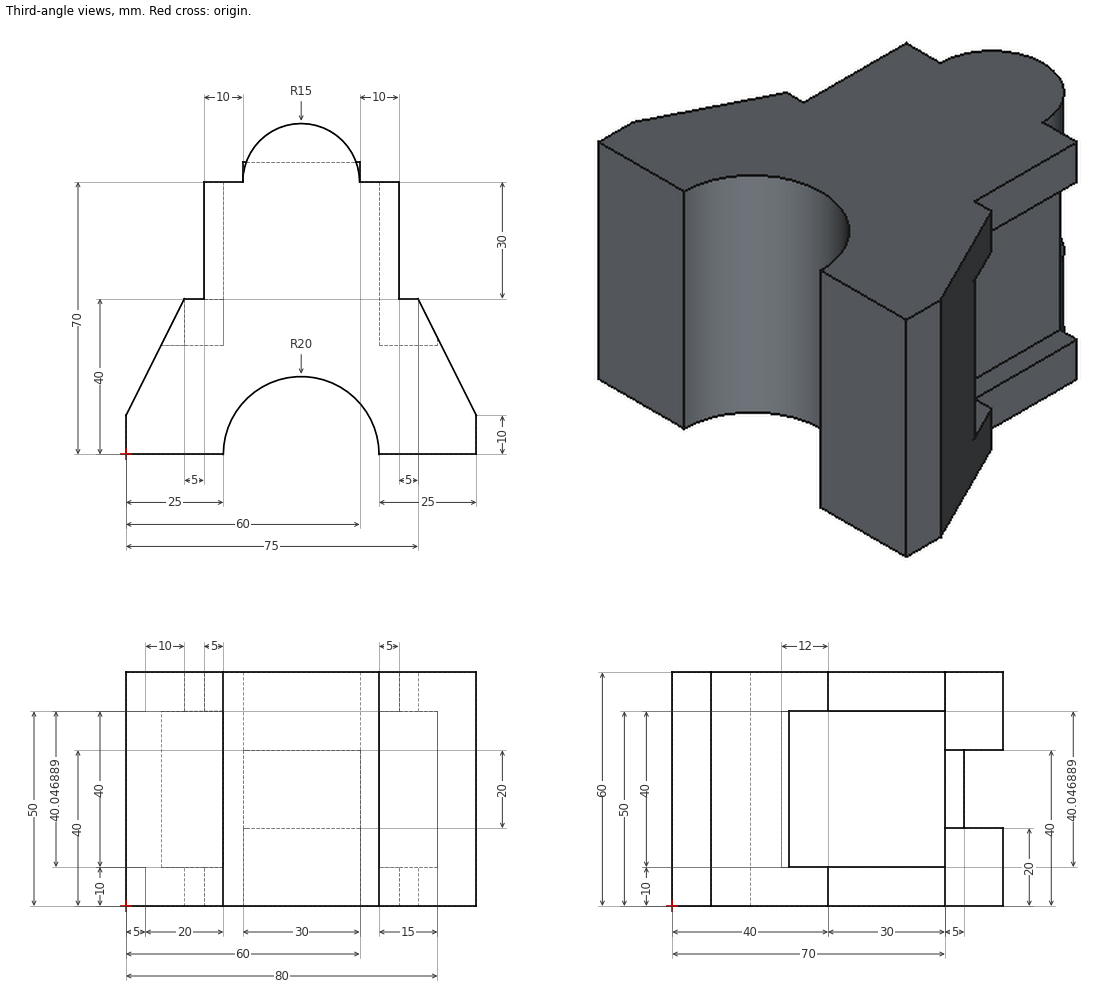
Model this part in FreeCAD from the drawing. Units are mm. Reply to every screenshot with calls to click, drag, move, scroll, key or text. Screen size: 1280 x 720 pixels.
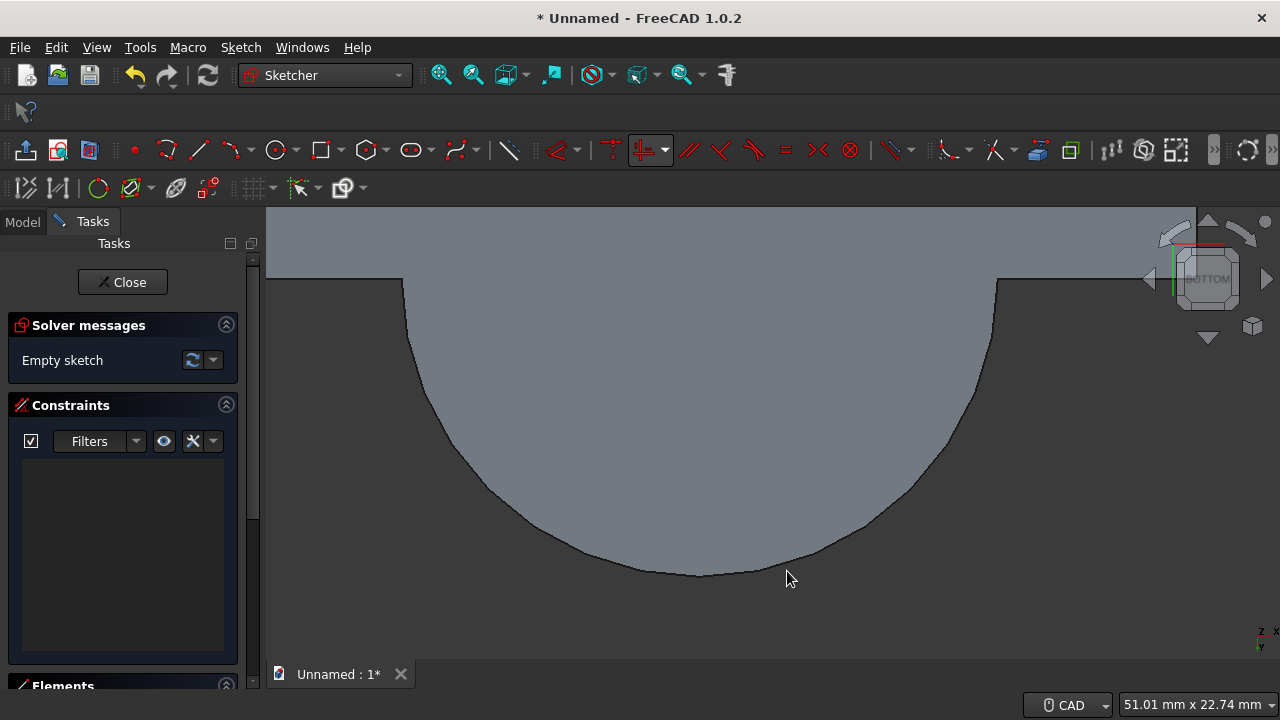
key(g)
key(l)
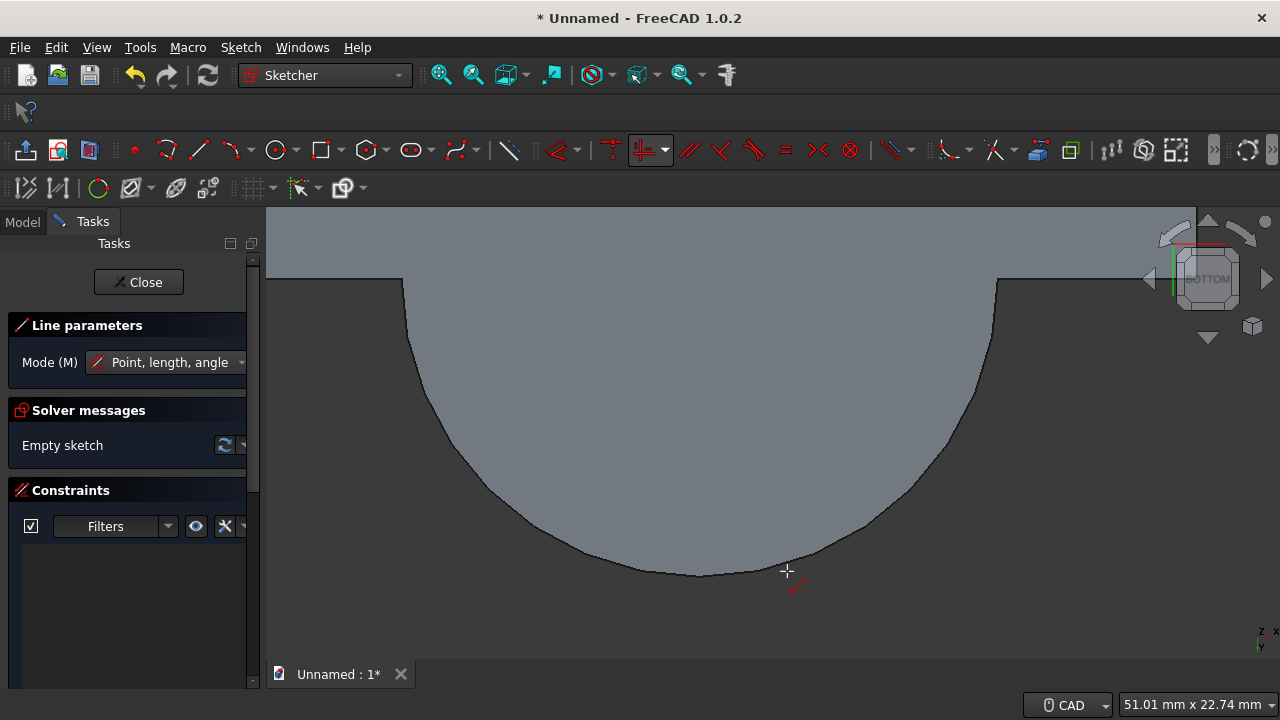
click(998, 279)
click(402, 279)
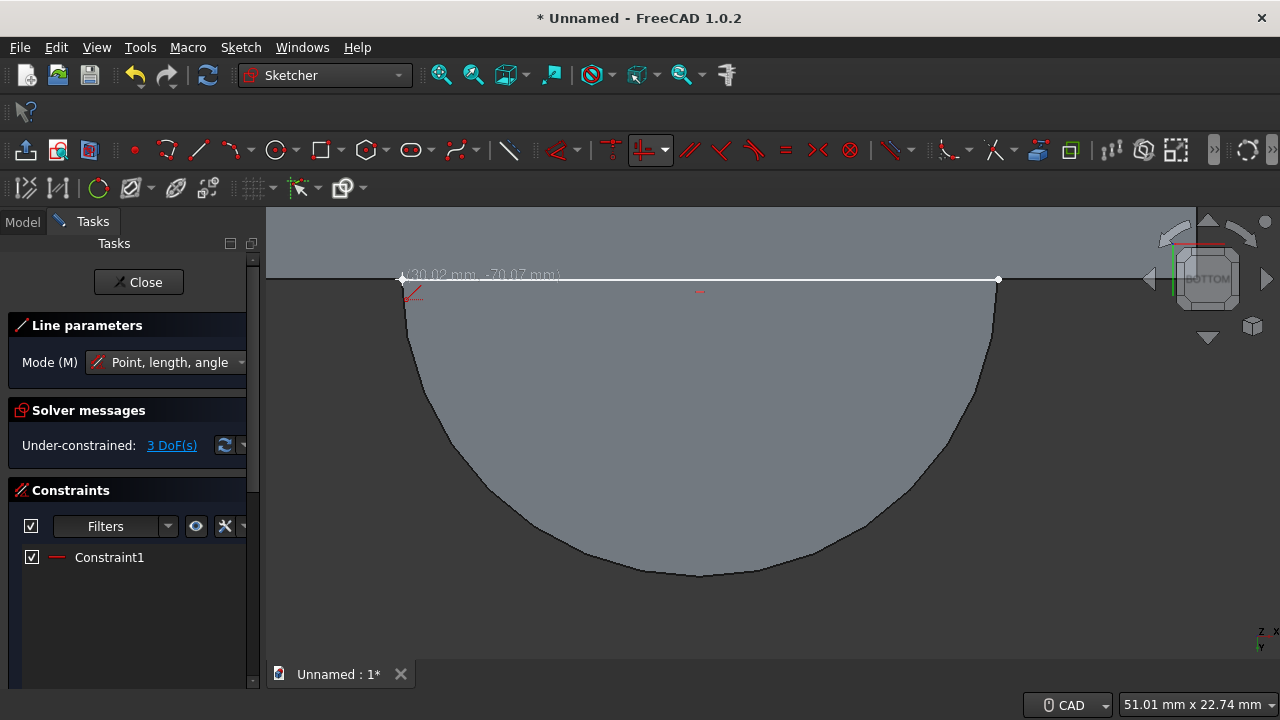
key(g)
key(3)
key(a)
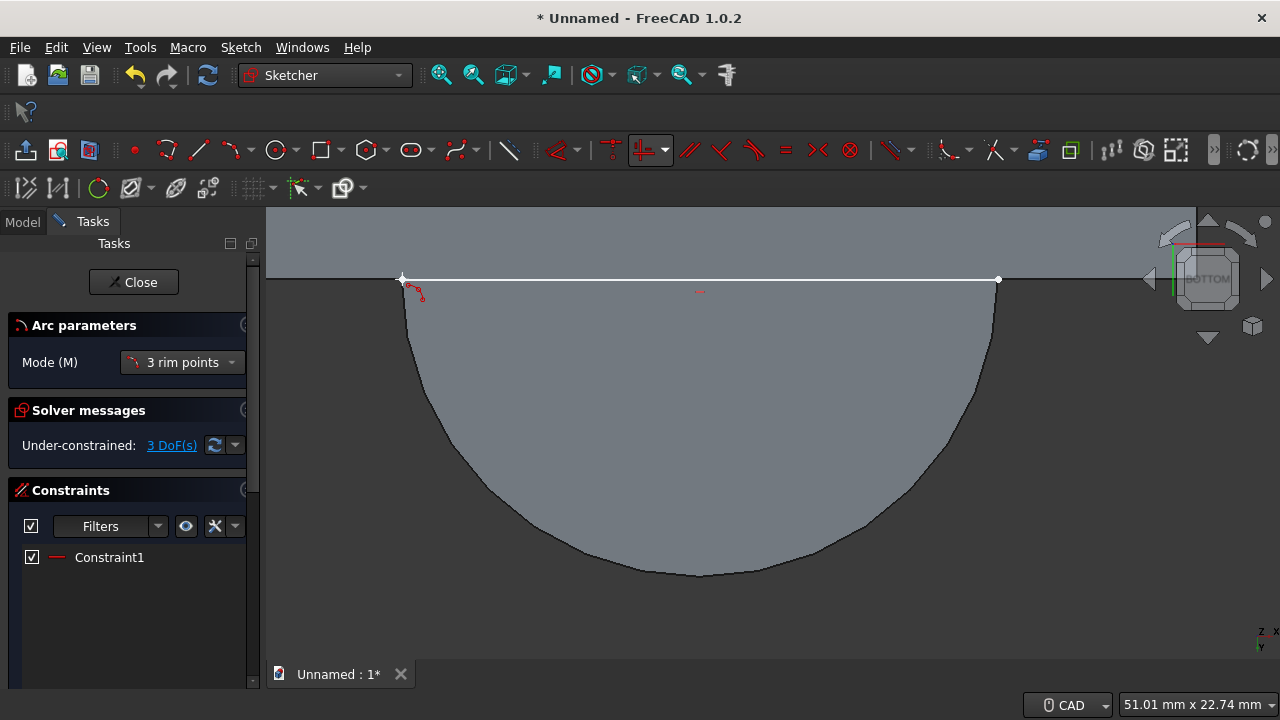
click(402, 280)
click(998, 280)
click(700, 577)
key(Escape)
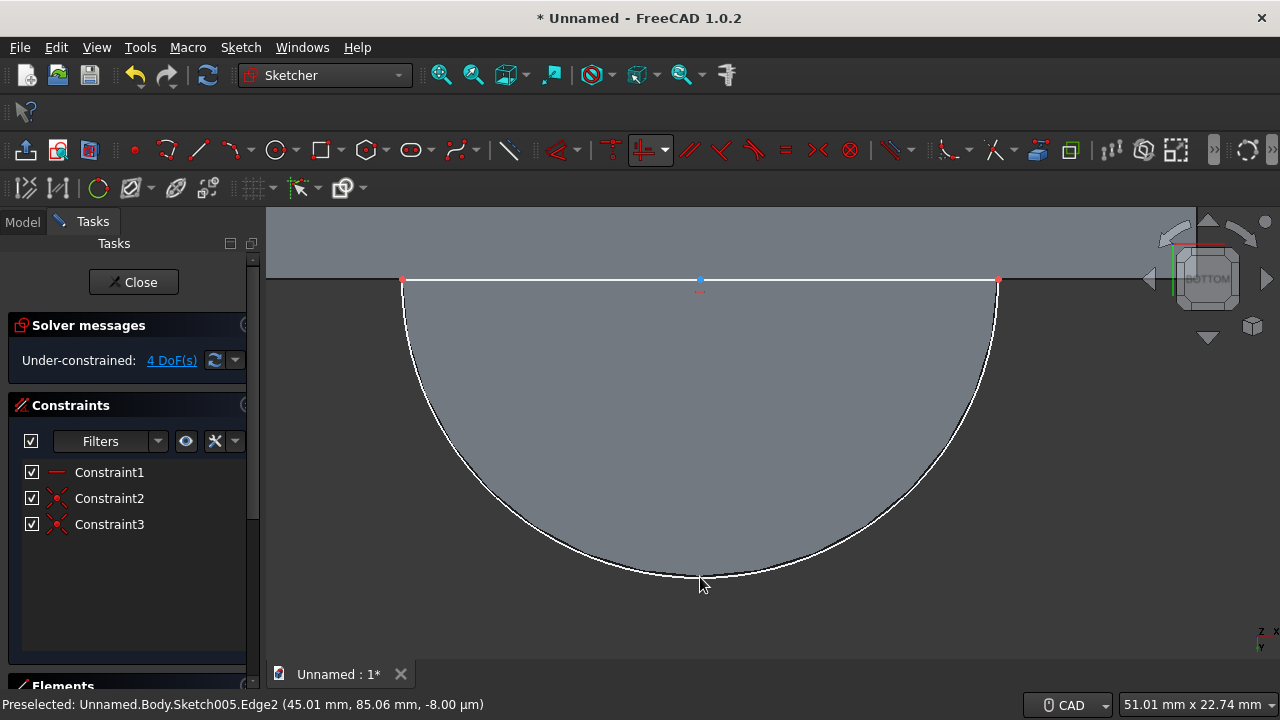
key(d)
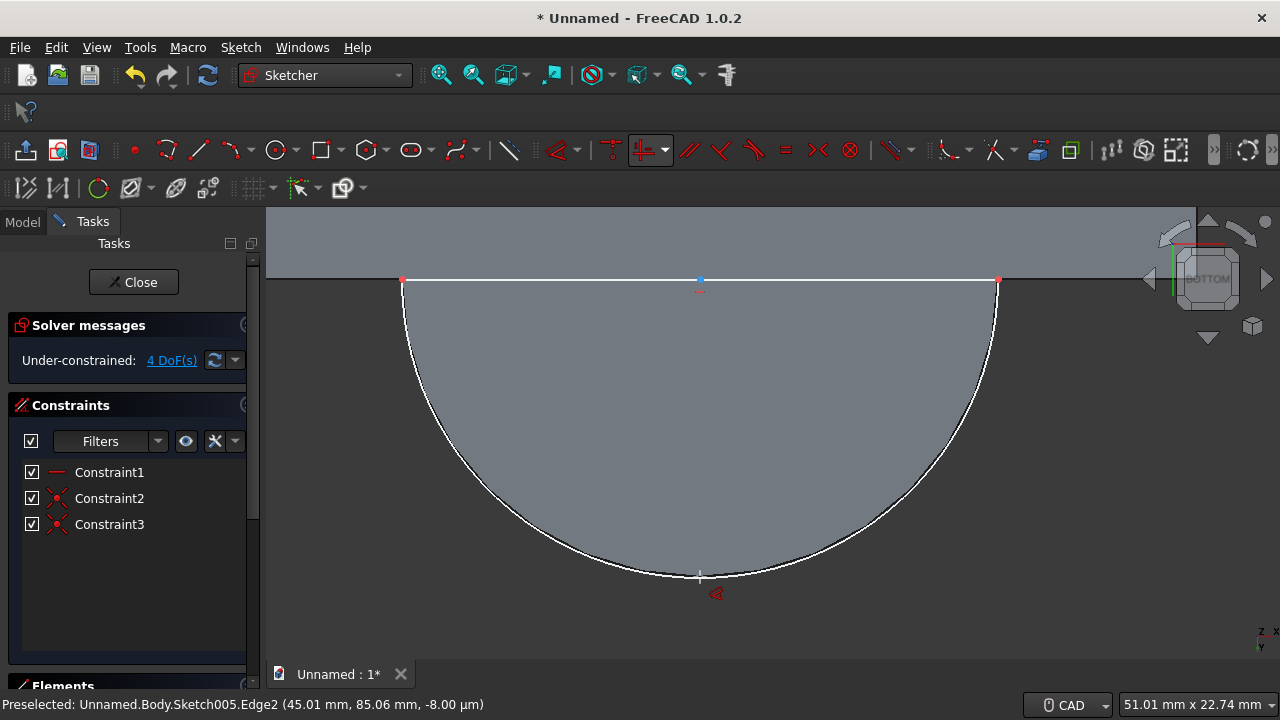
click(525, 521)
click(506, 547)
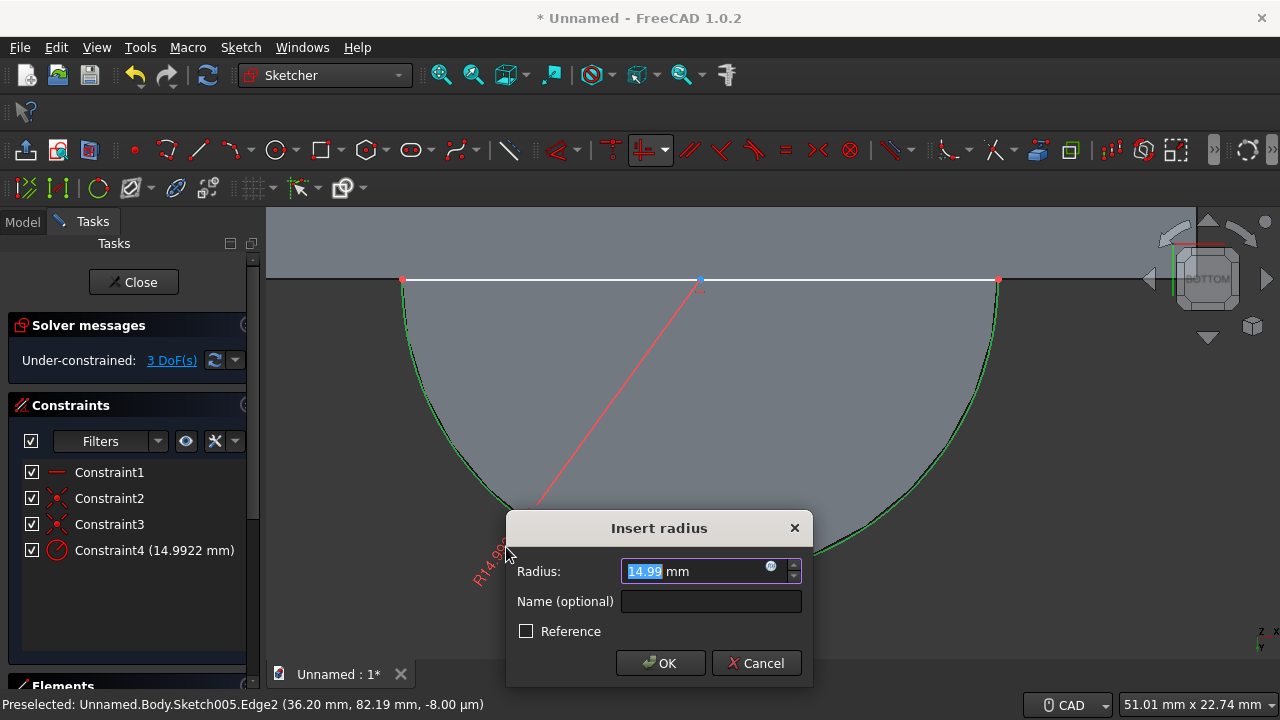
text(15)
key(Return)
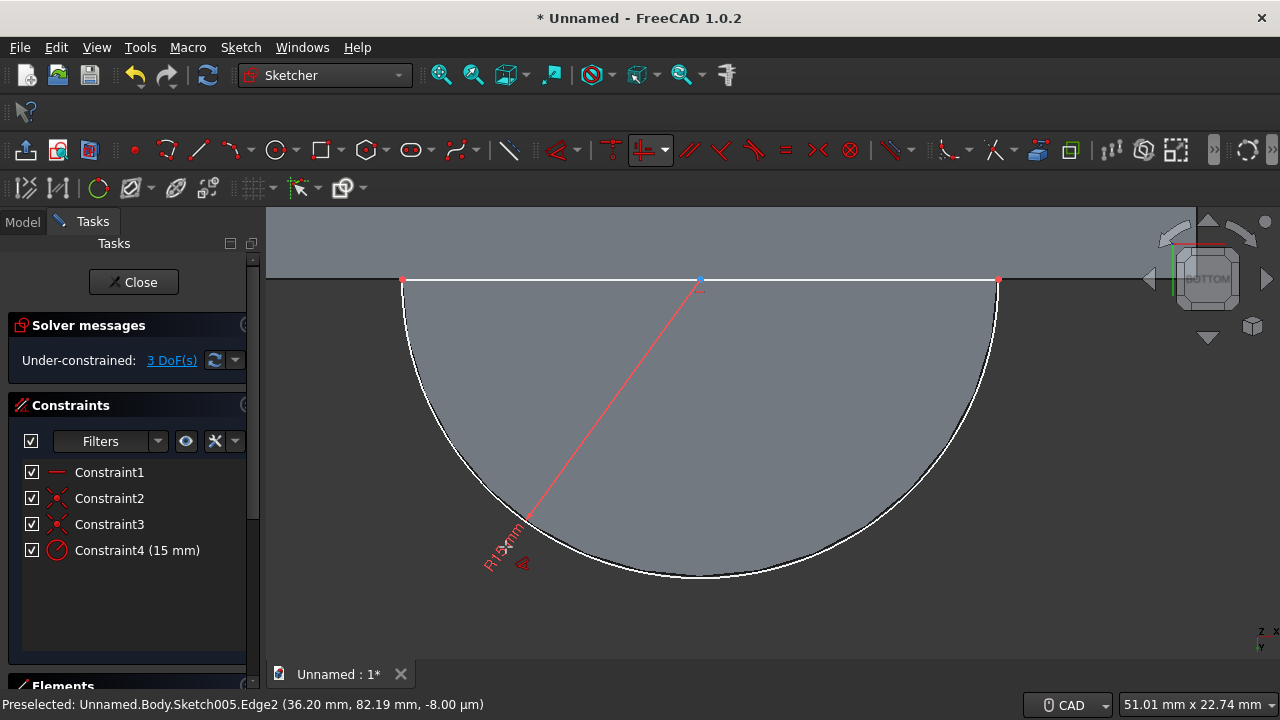
click(998, 280)
click(646, 314)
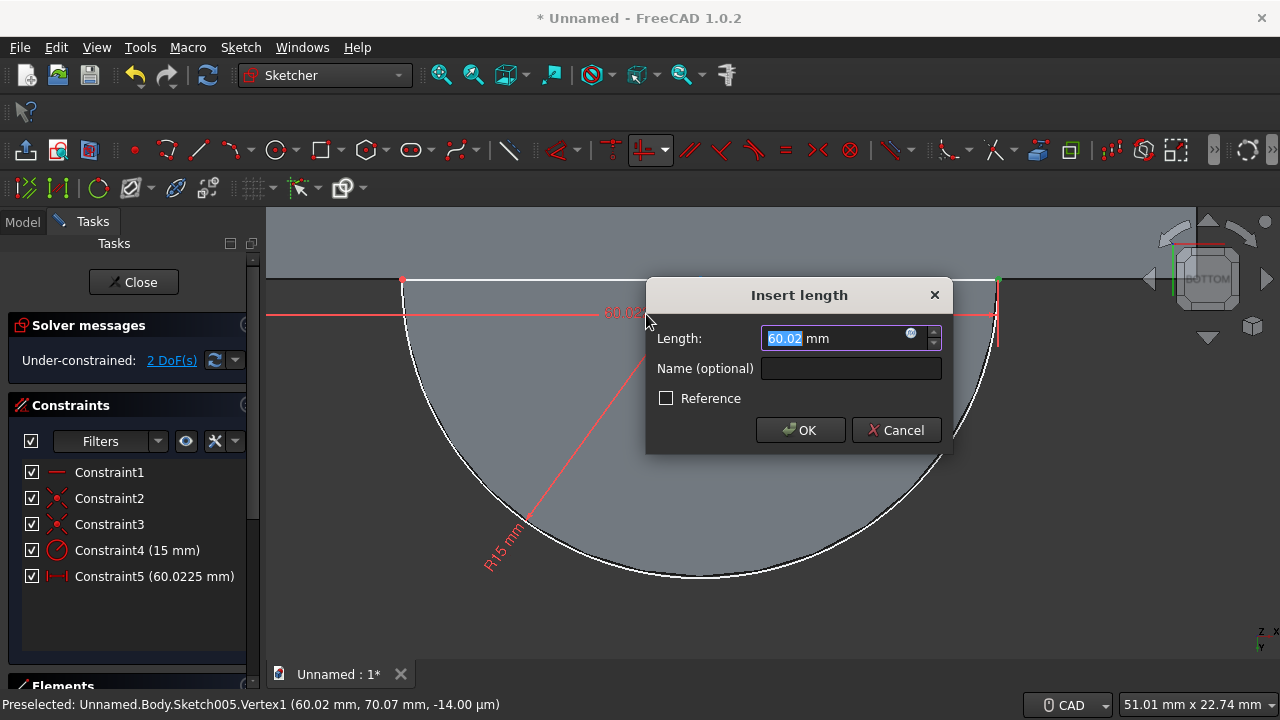
text(60)
key(Return)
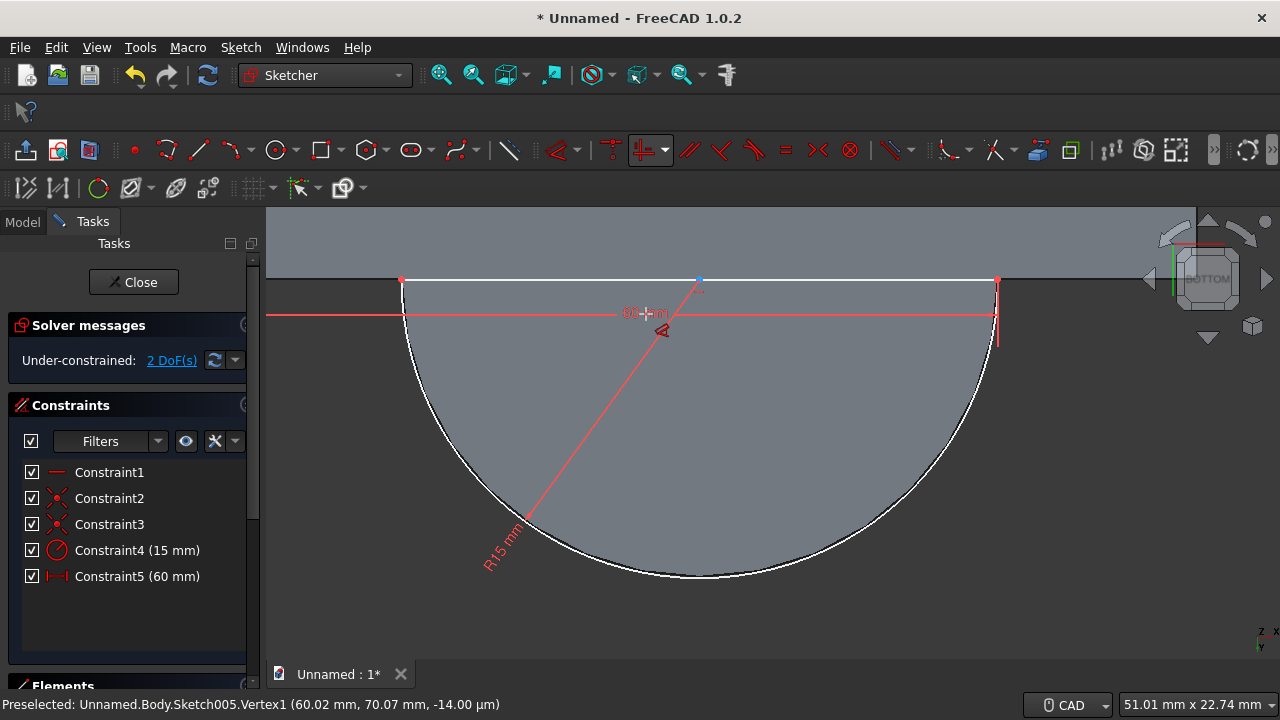
click(998, 280)
click(1032, 258)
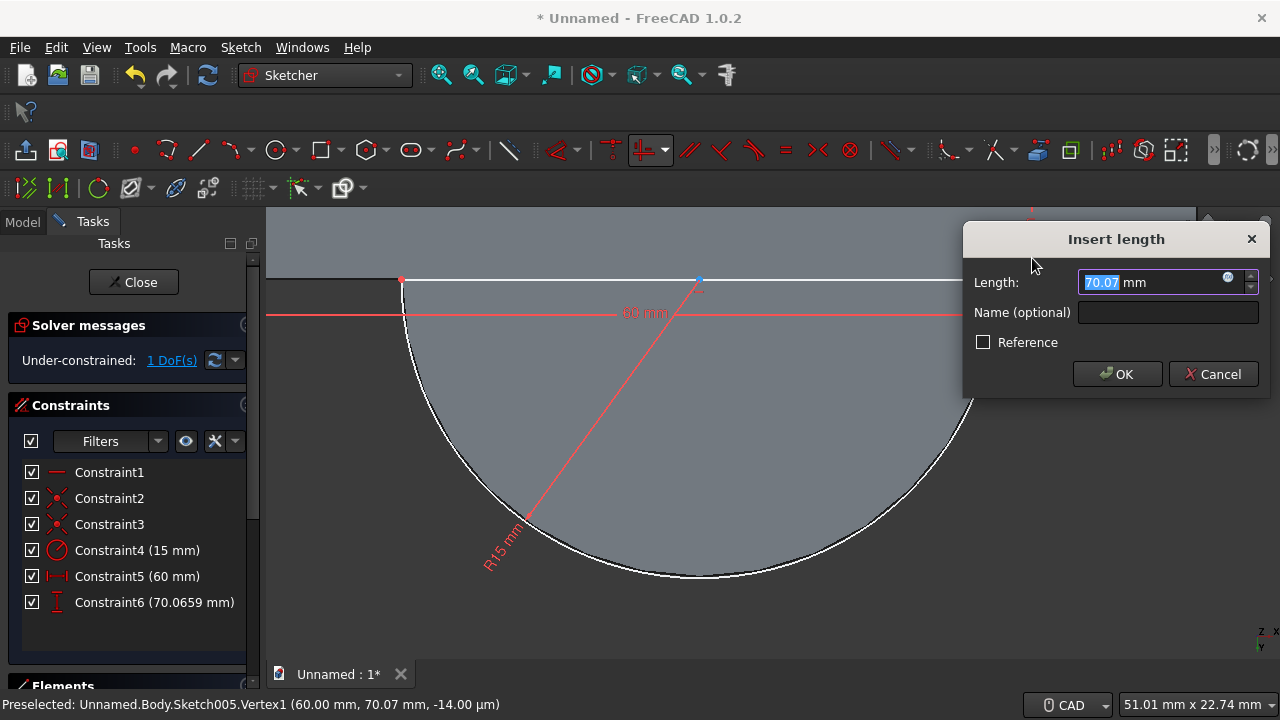
text(70)
key(Return)